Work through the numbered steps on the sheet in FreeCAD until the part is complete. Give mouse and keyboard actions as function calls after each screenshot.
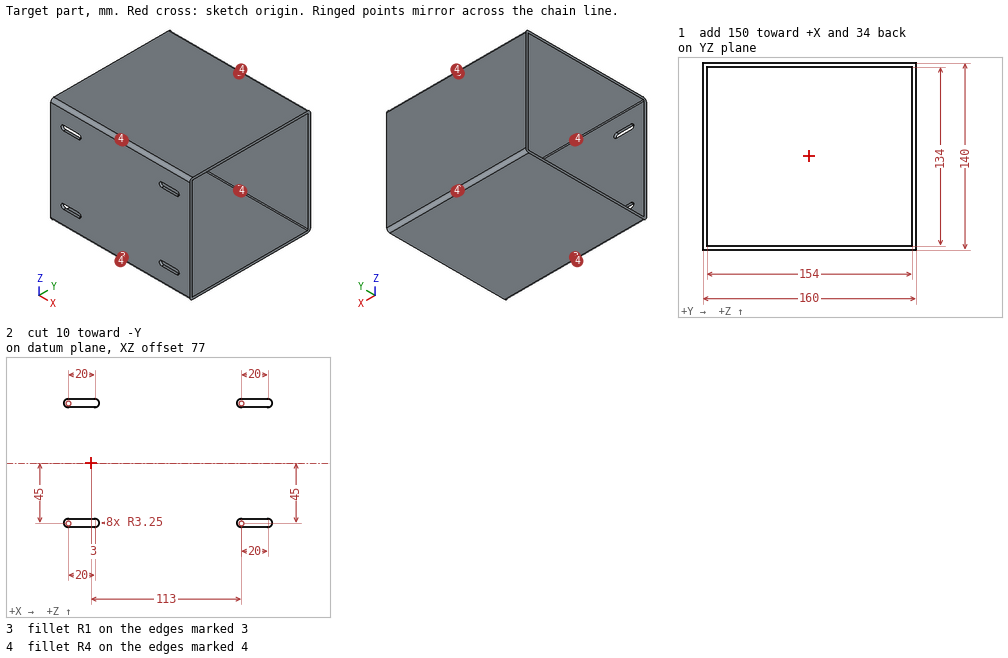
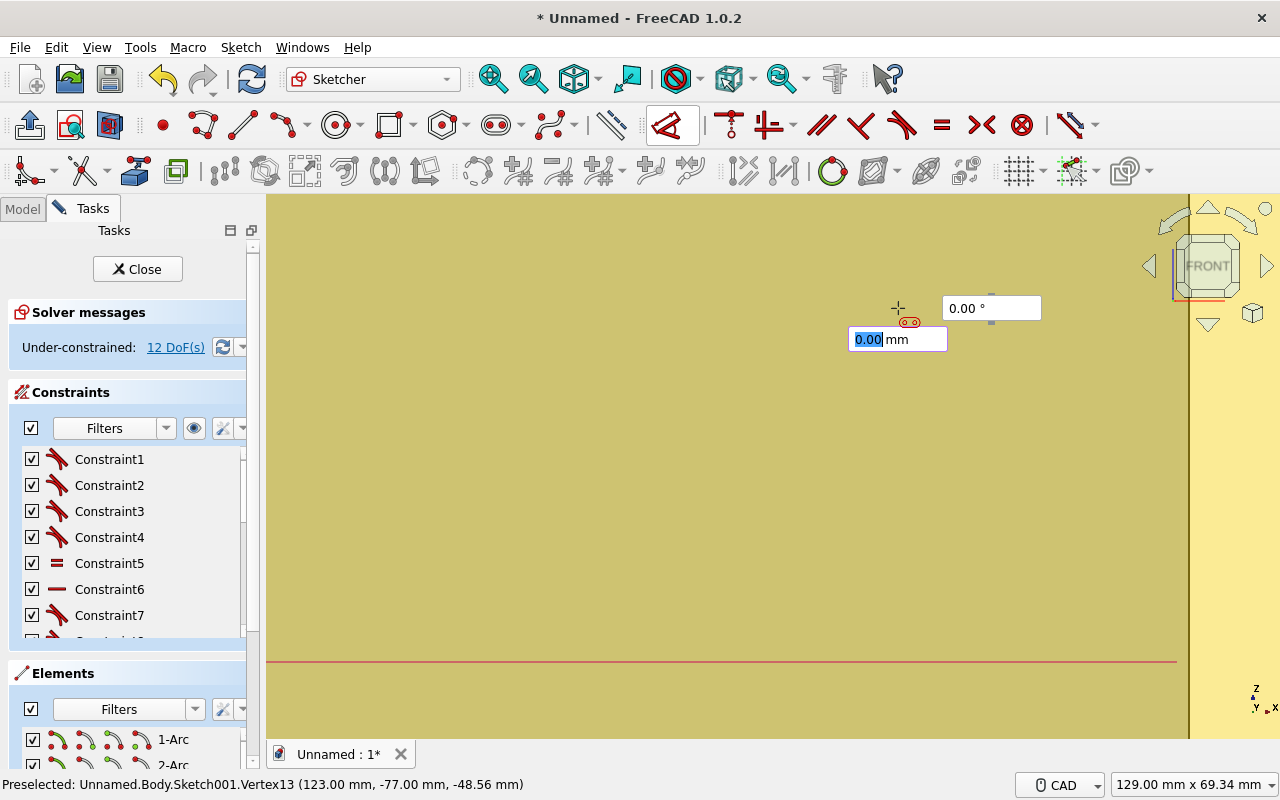
click(1056, 308)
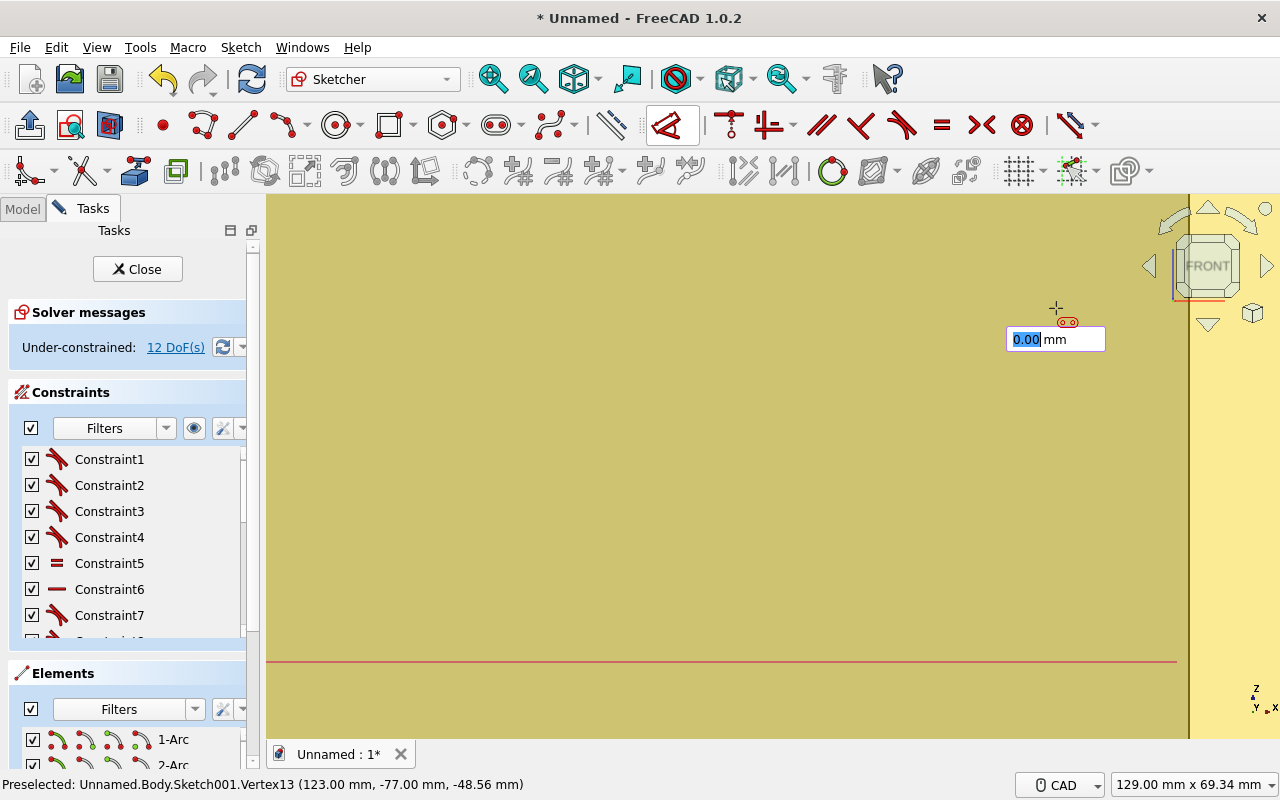
click(977, 282)
key(Escape)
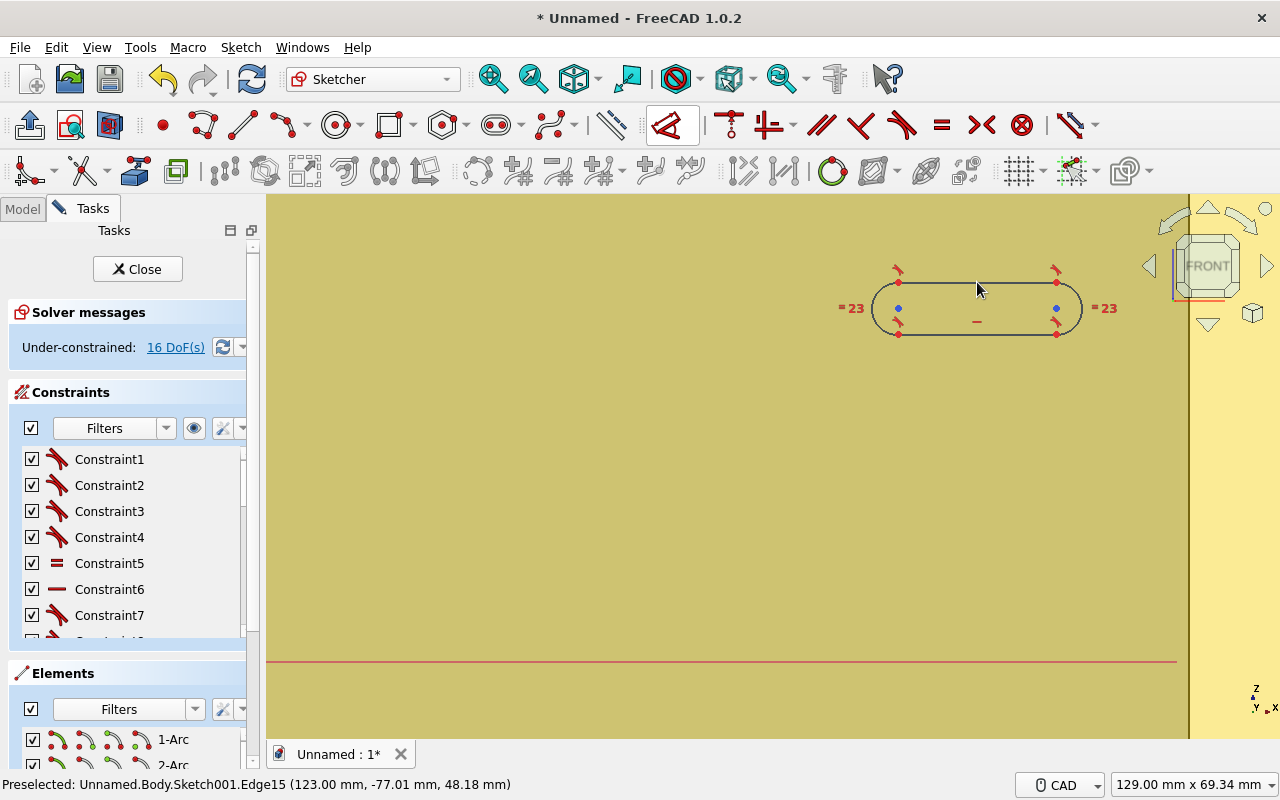
scroll(899, 307, down, 4)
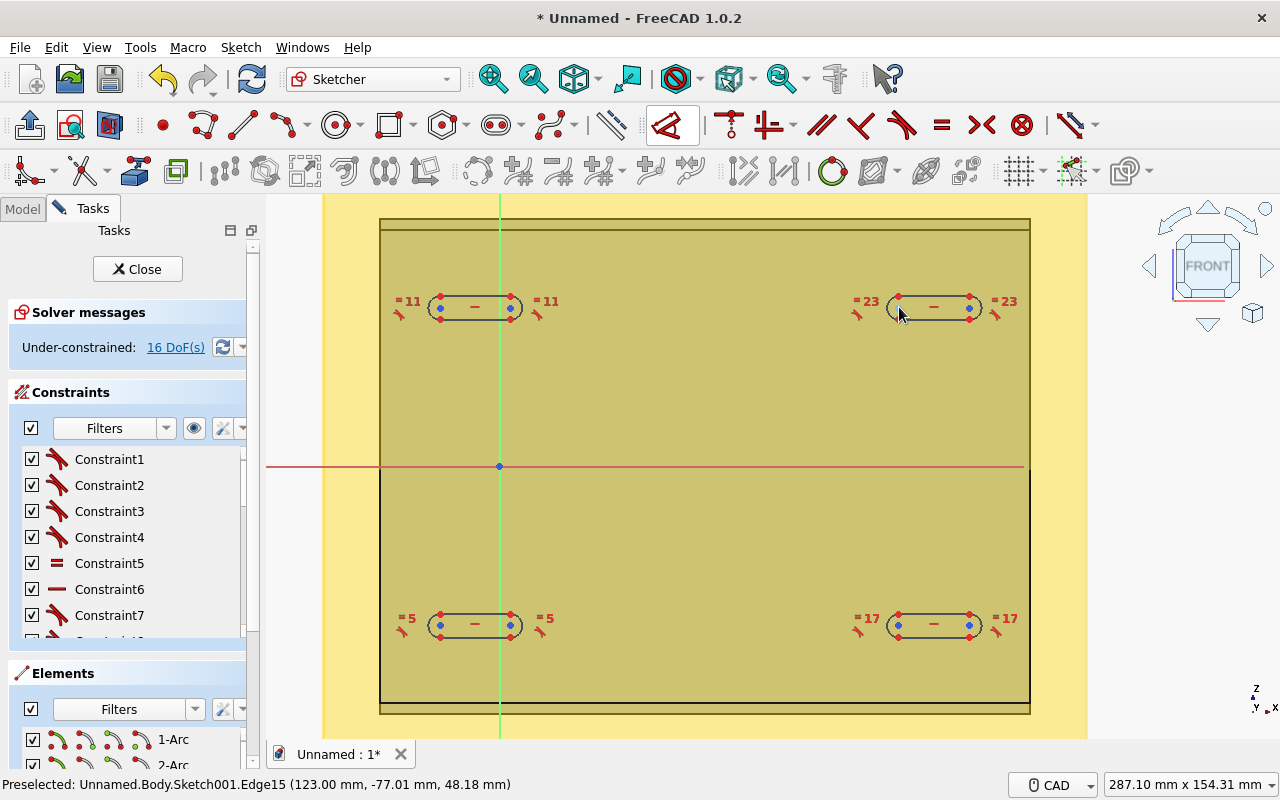
scroll(431, 619, up, 2)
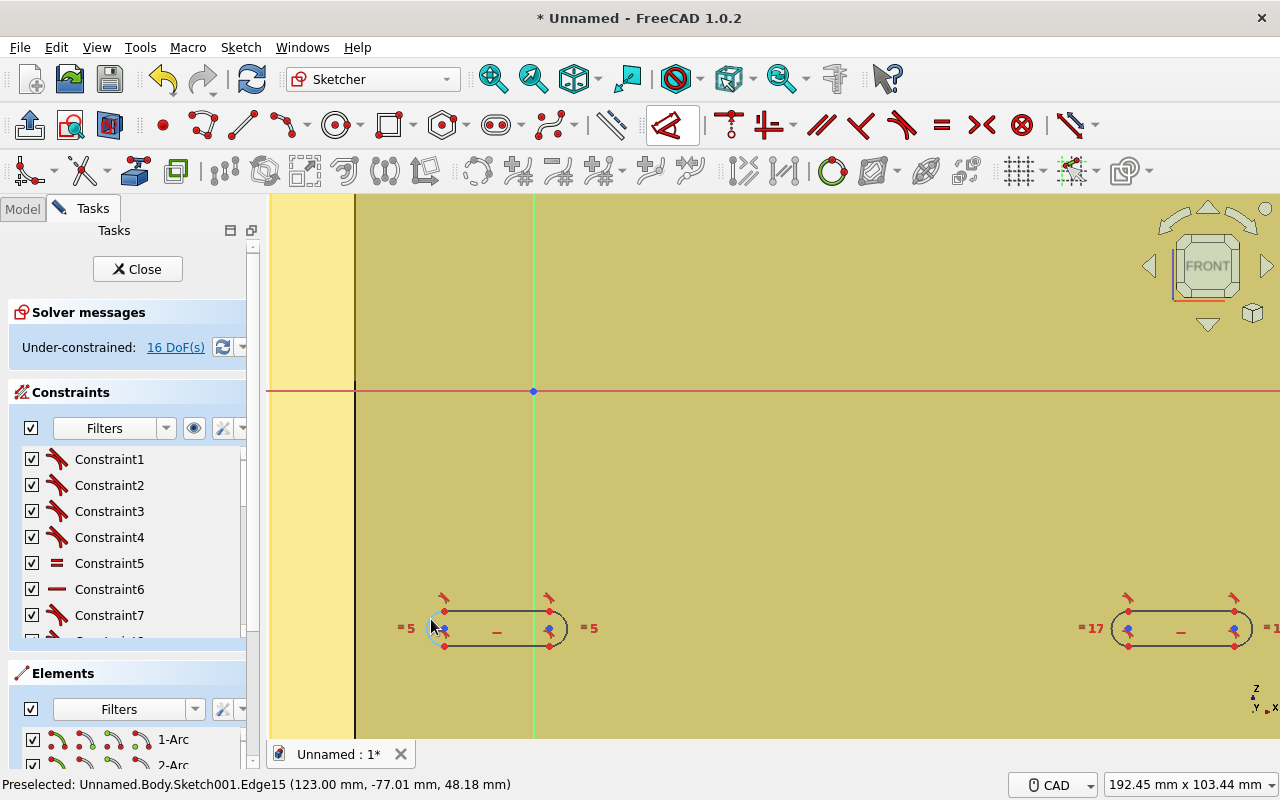
click(430, 619)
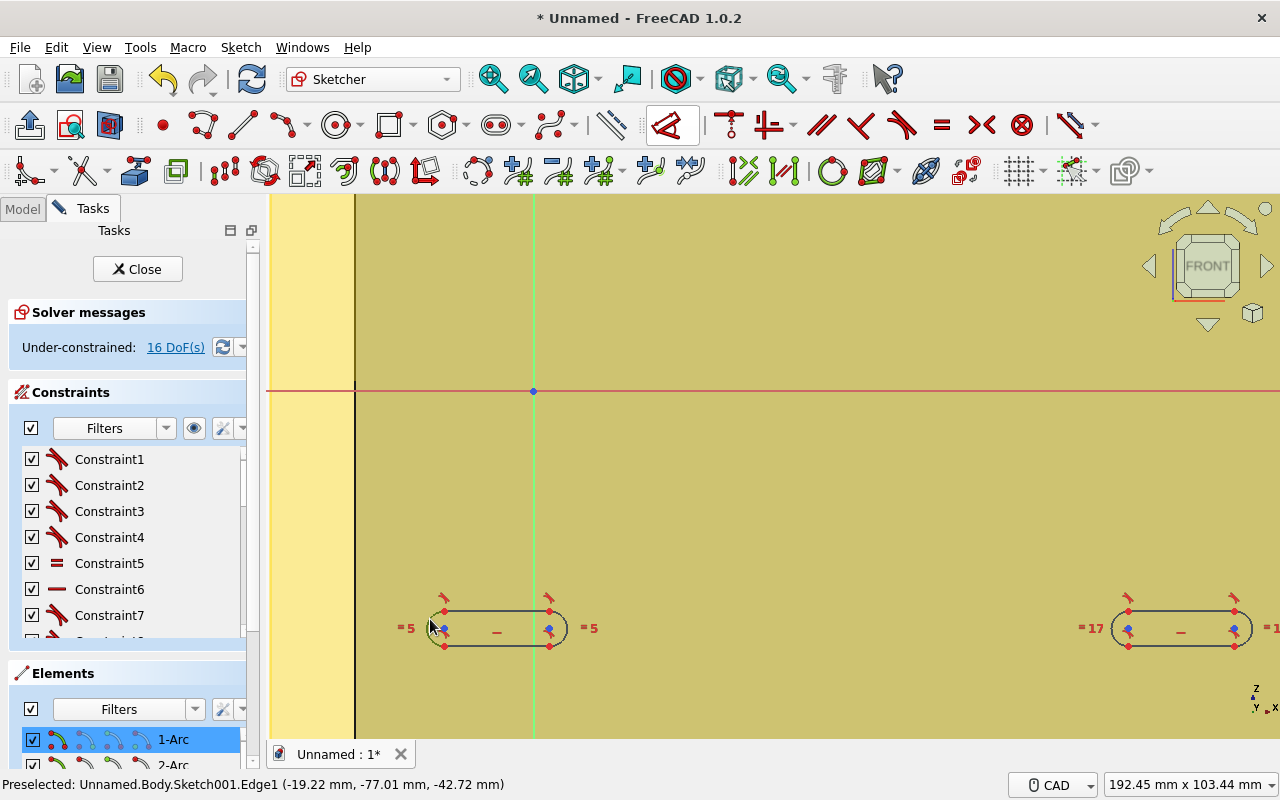
scroll(430, 620, down, 2)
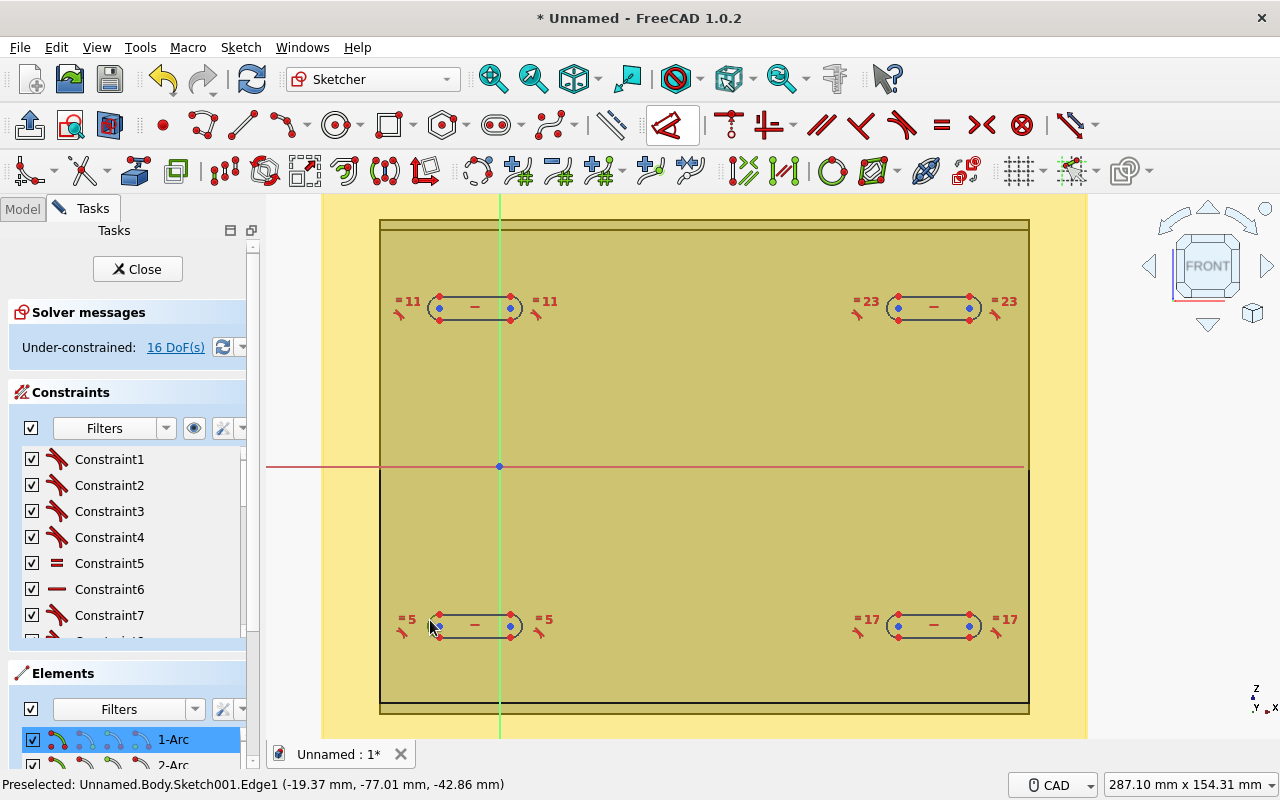
scroll(430, 301, up, 2)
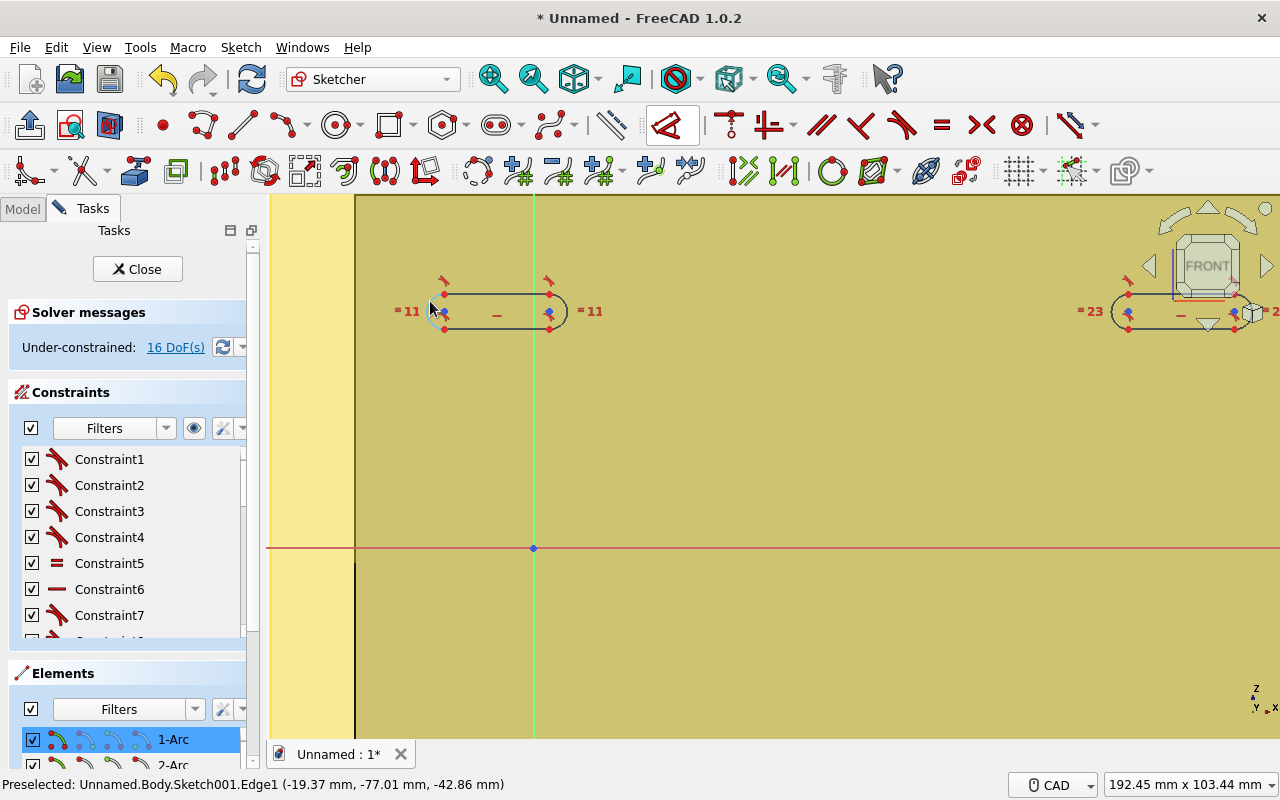
click(430, 302)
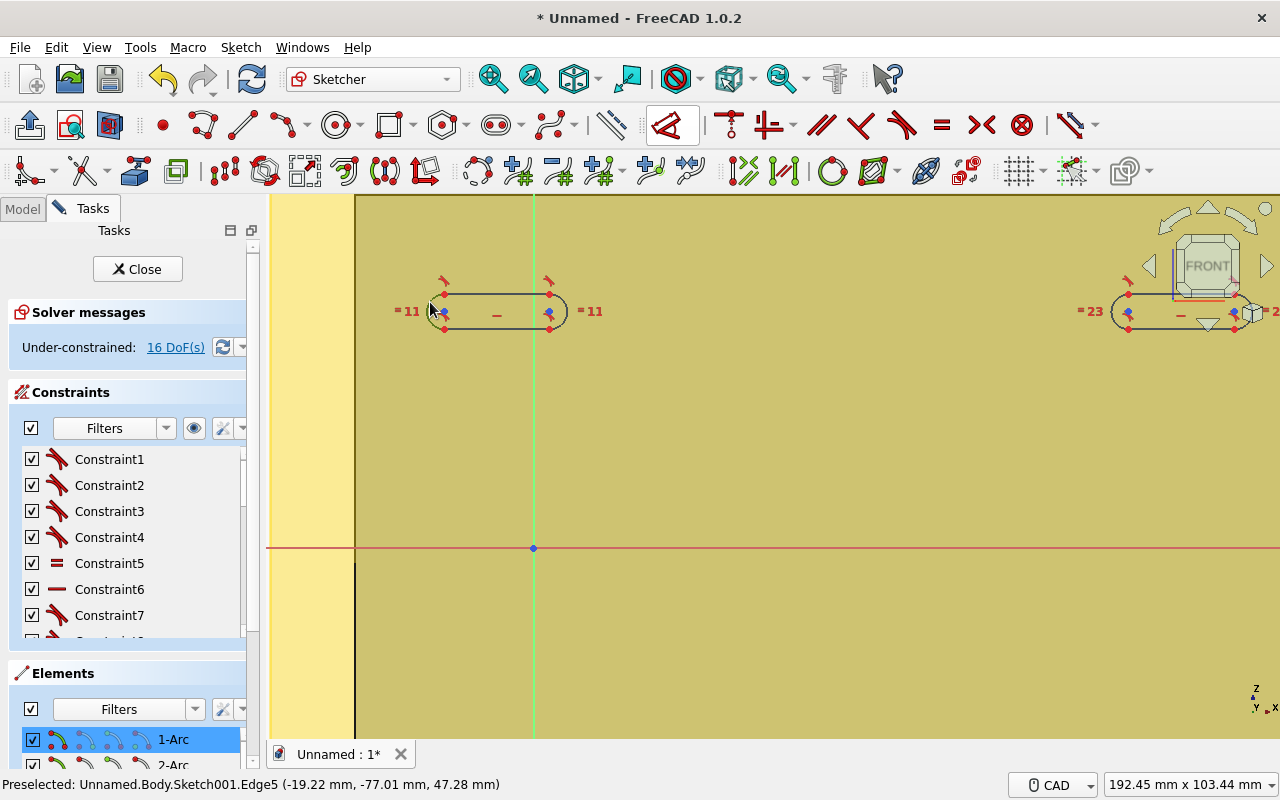
scroll(430, 300, down, 2)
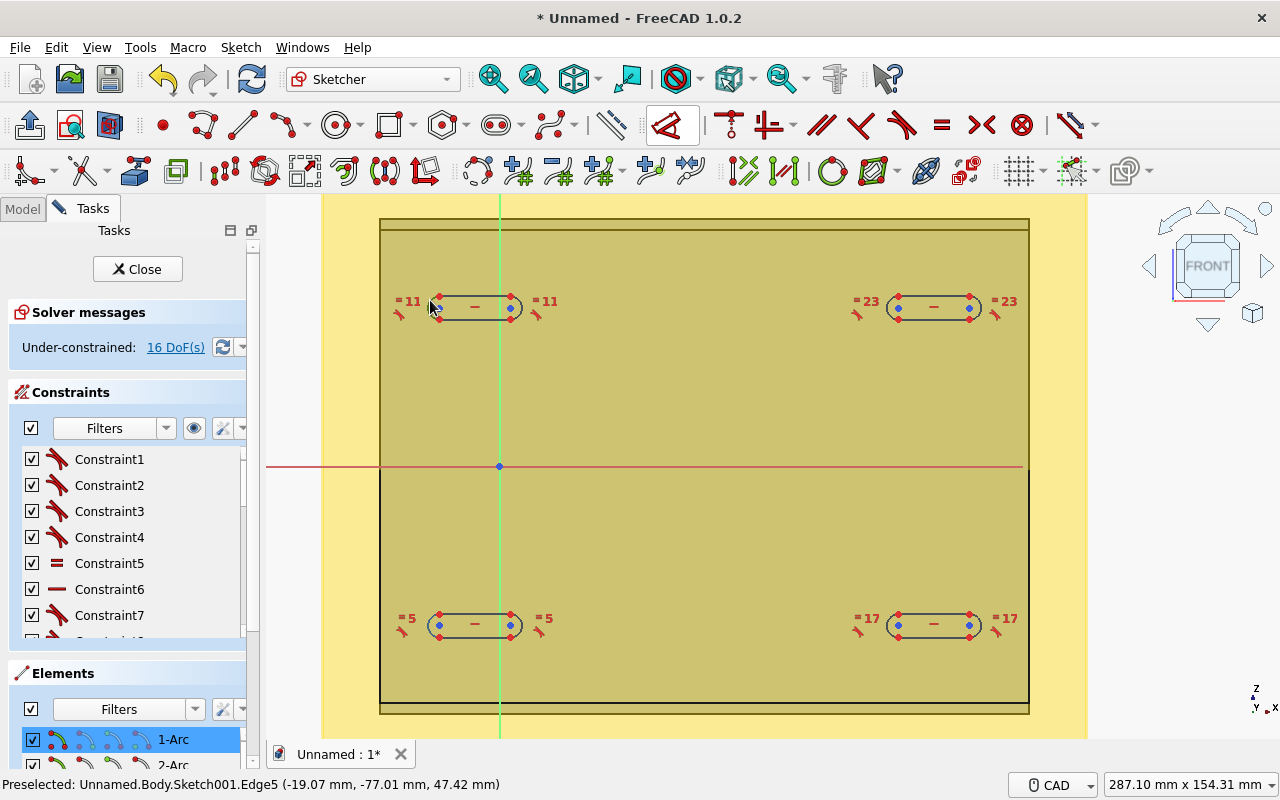
scroll(889, 619, up, 2)